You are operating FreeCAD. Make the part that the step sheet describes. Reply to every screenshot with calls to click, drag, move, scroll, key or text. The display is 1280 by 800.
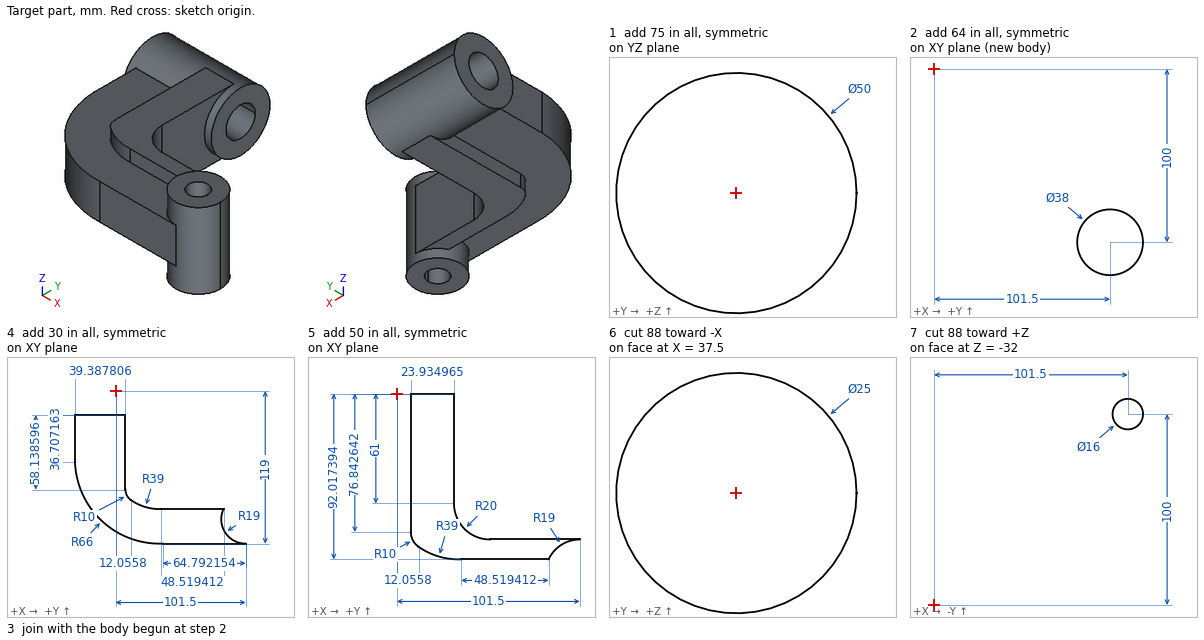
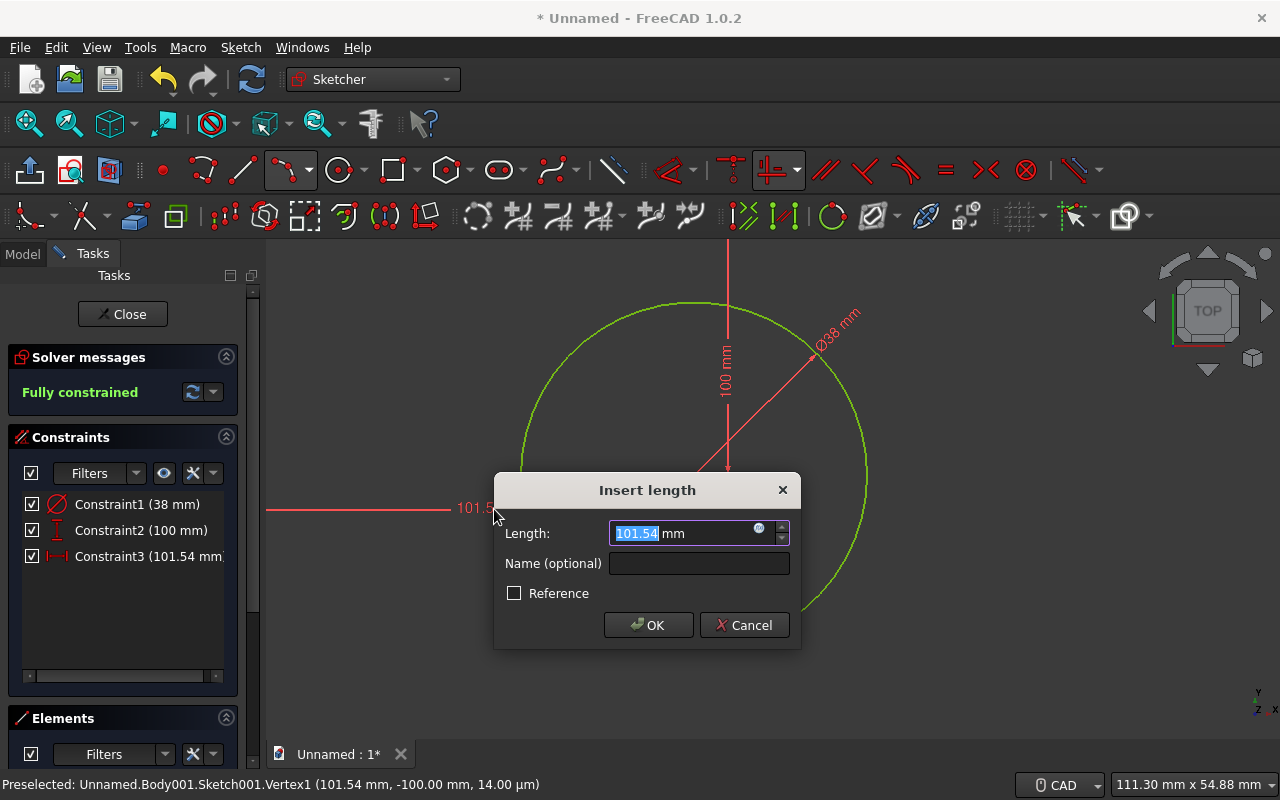
text(101.5)
key(Return)
key(Escape)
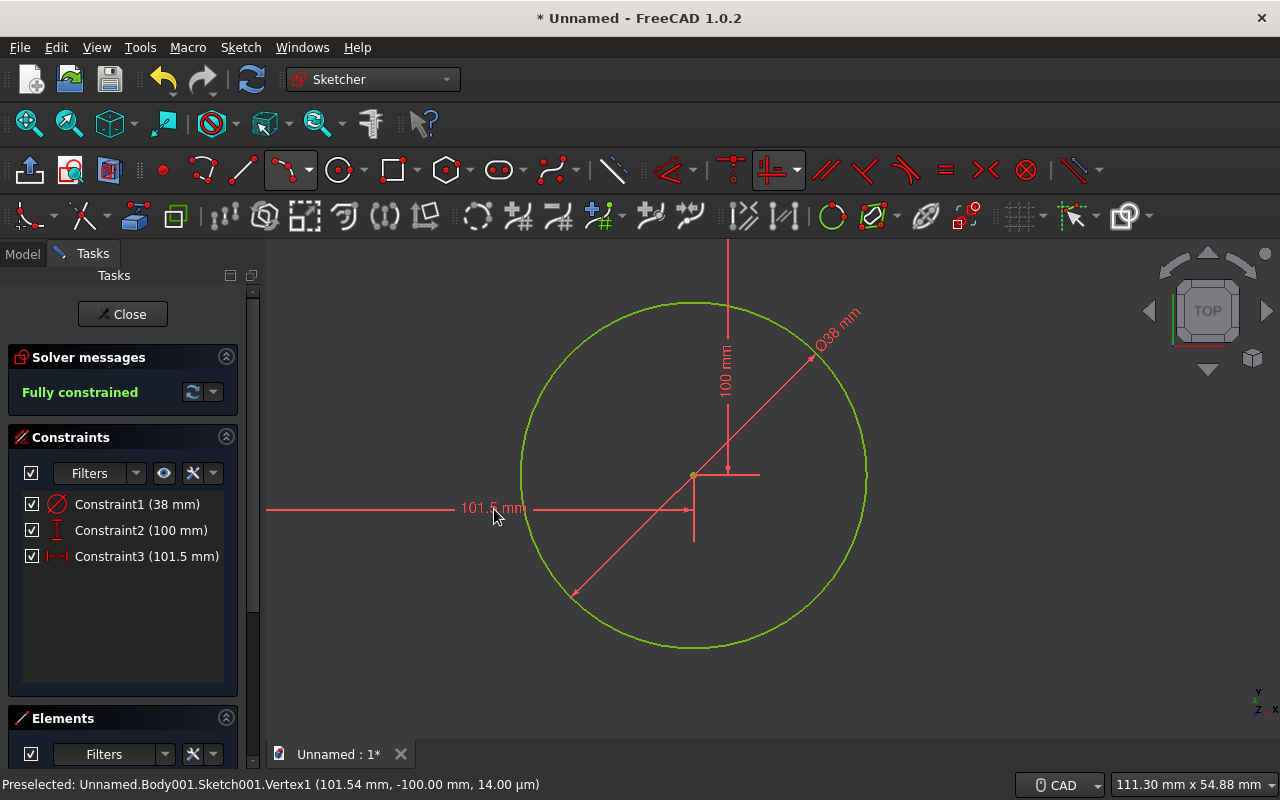
click(123, 314)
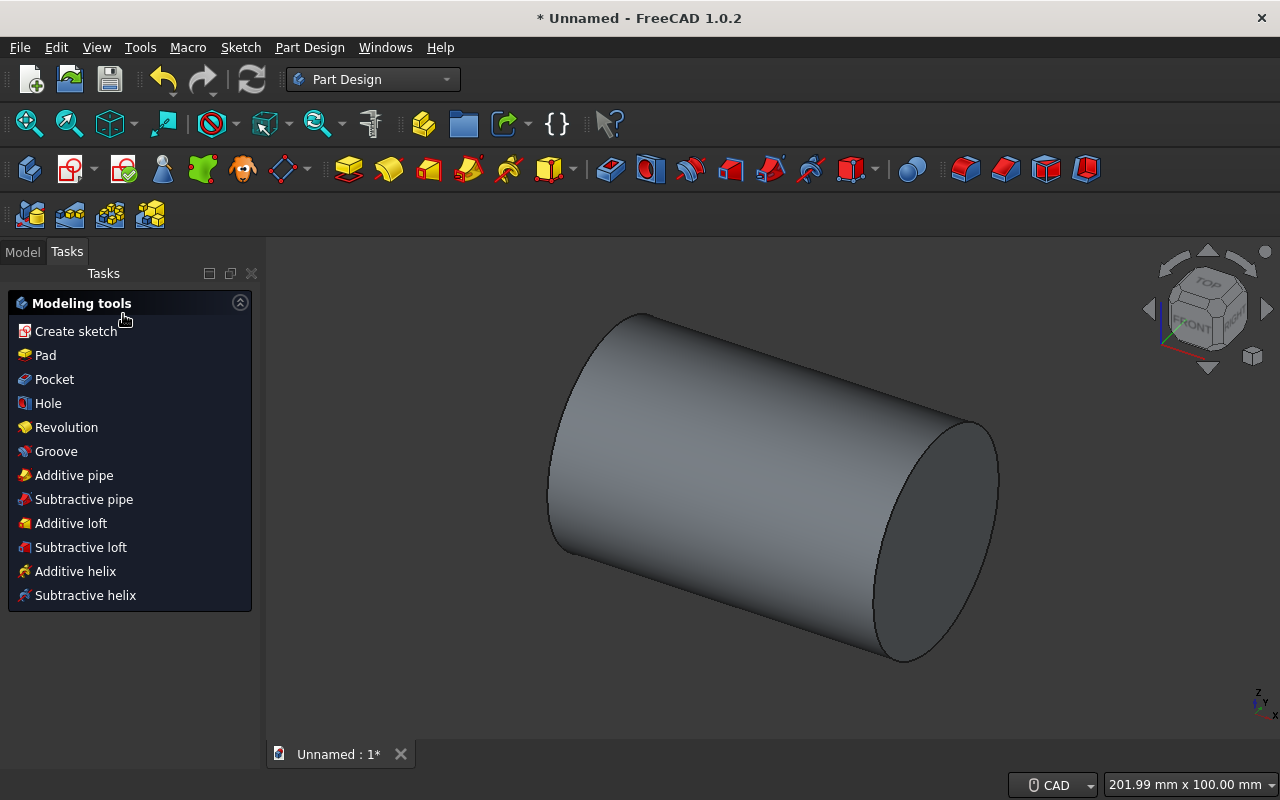
click(350, 170)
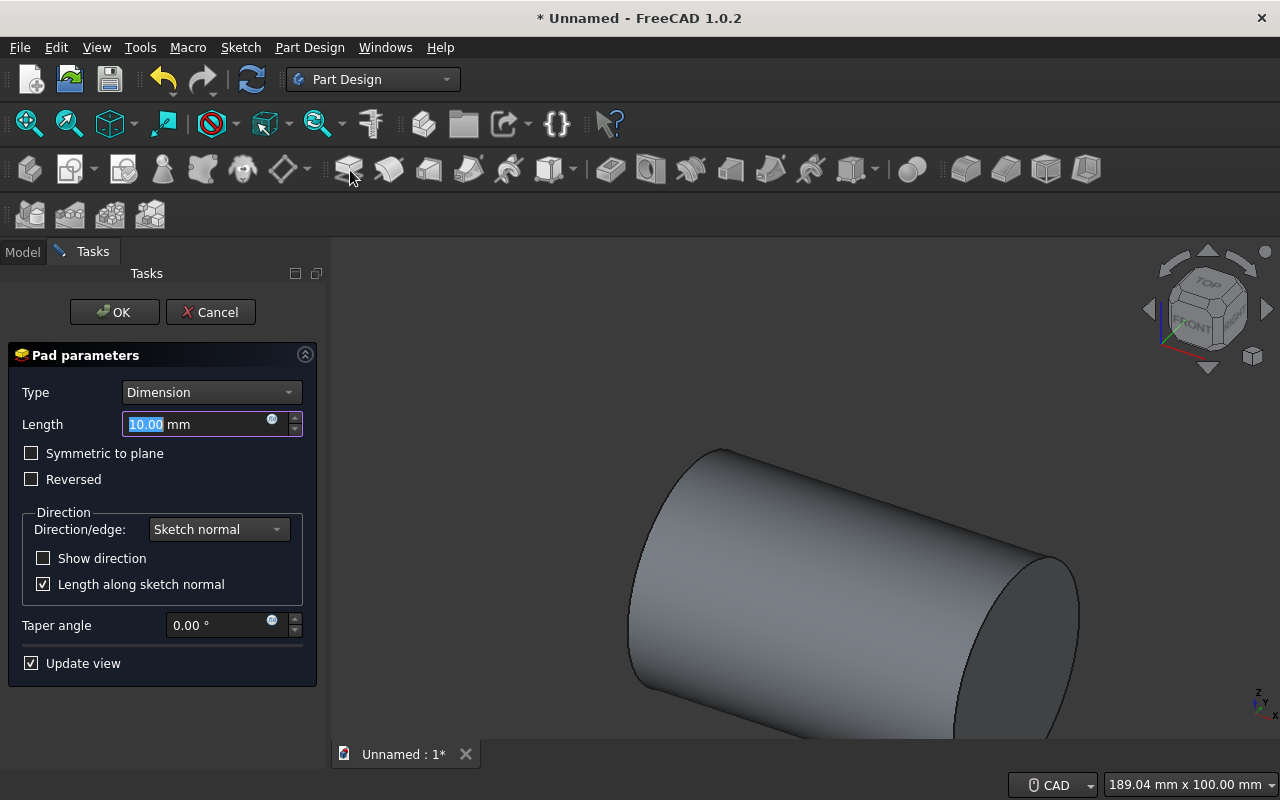
text(64)
key(Tab)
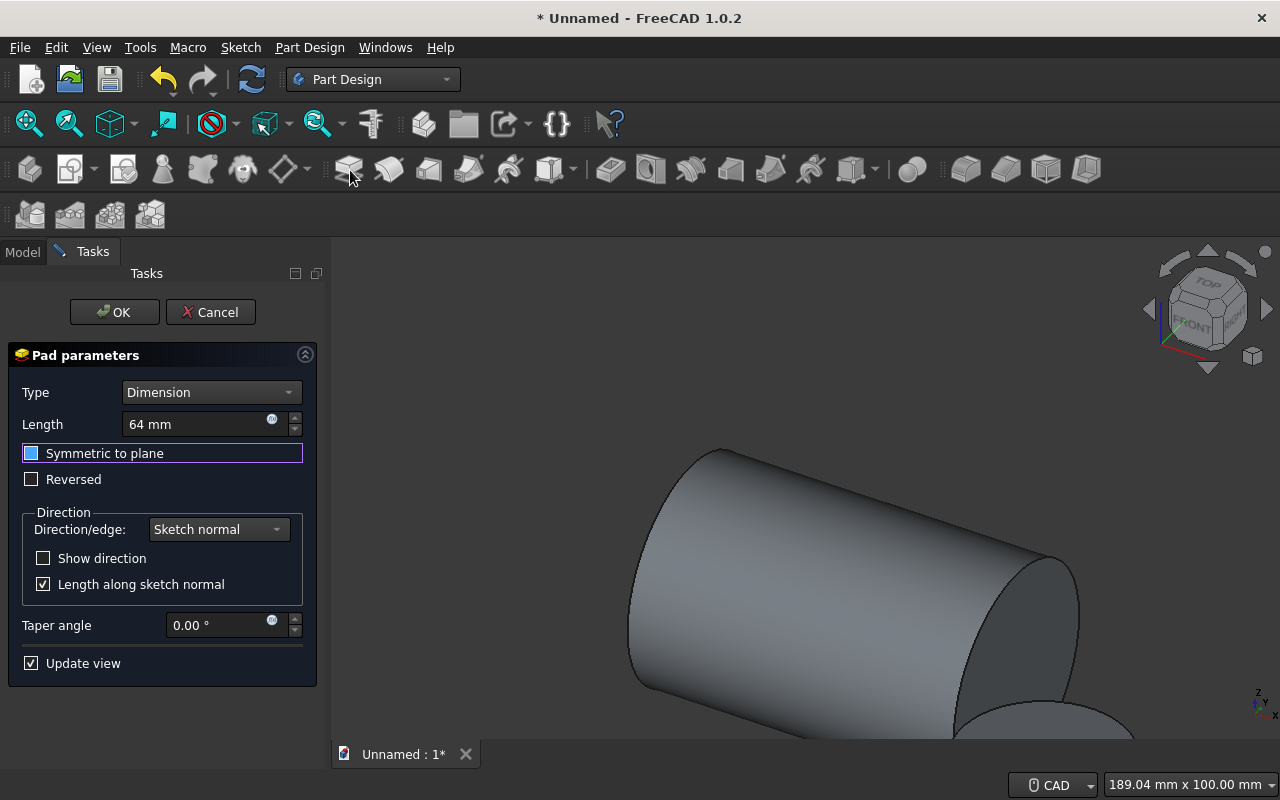
click(30, 453)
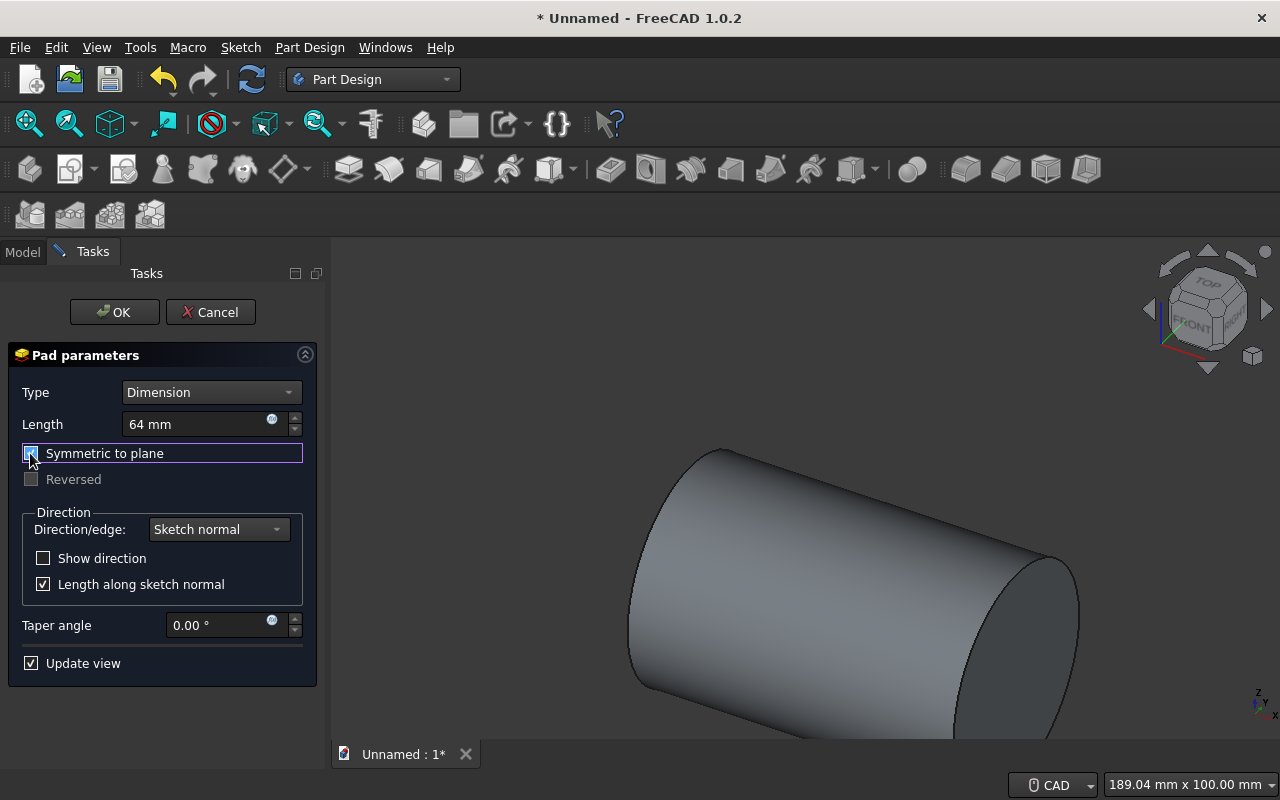
click(115, 312)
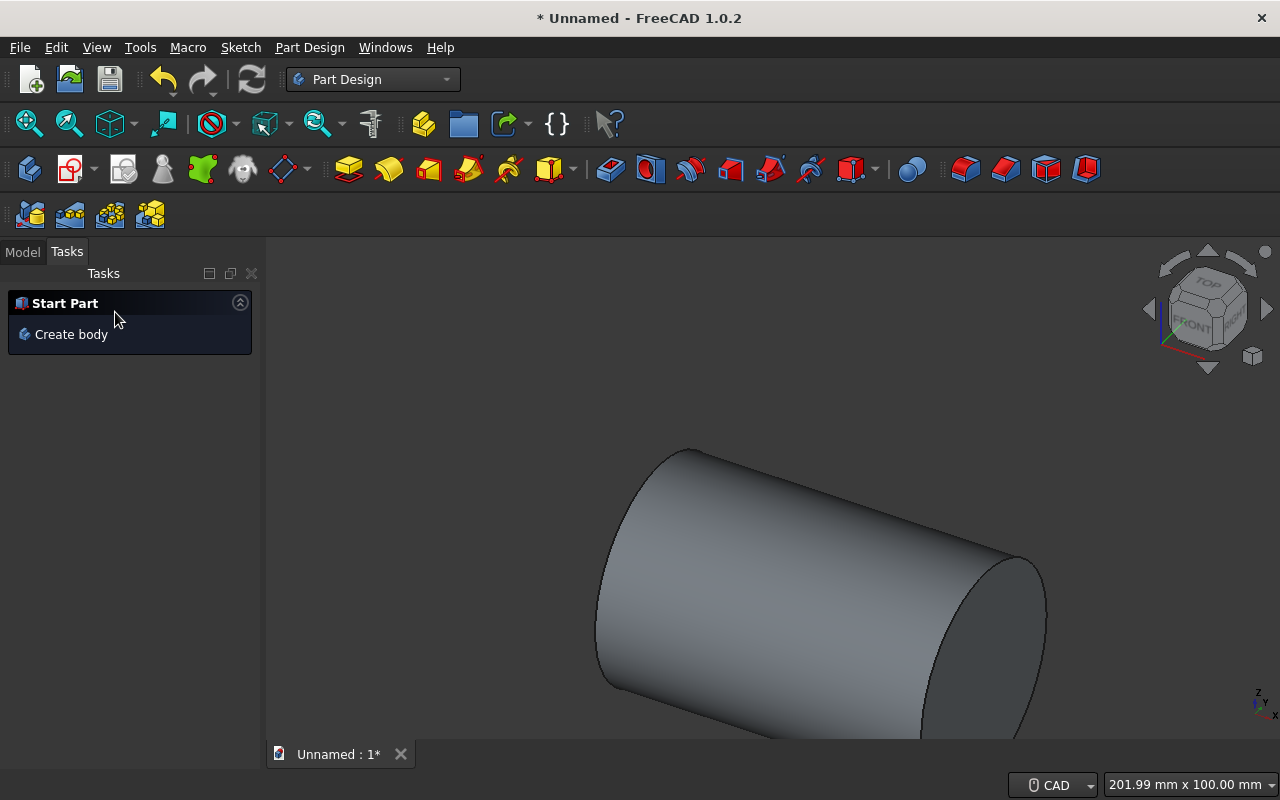
key(v)
key(f)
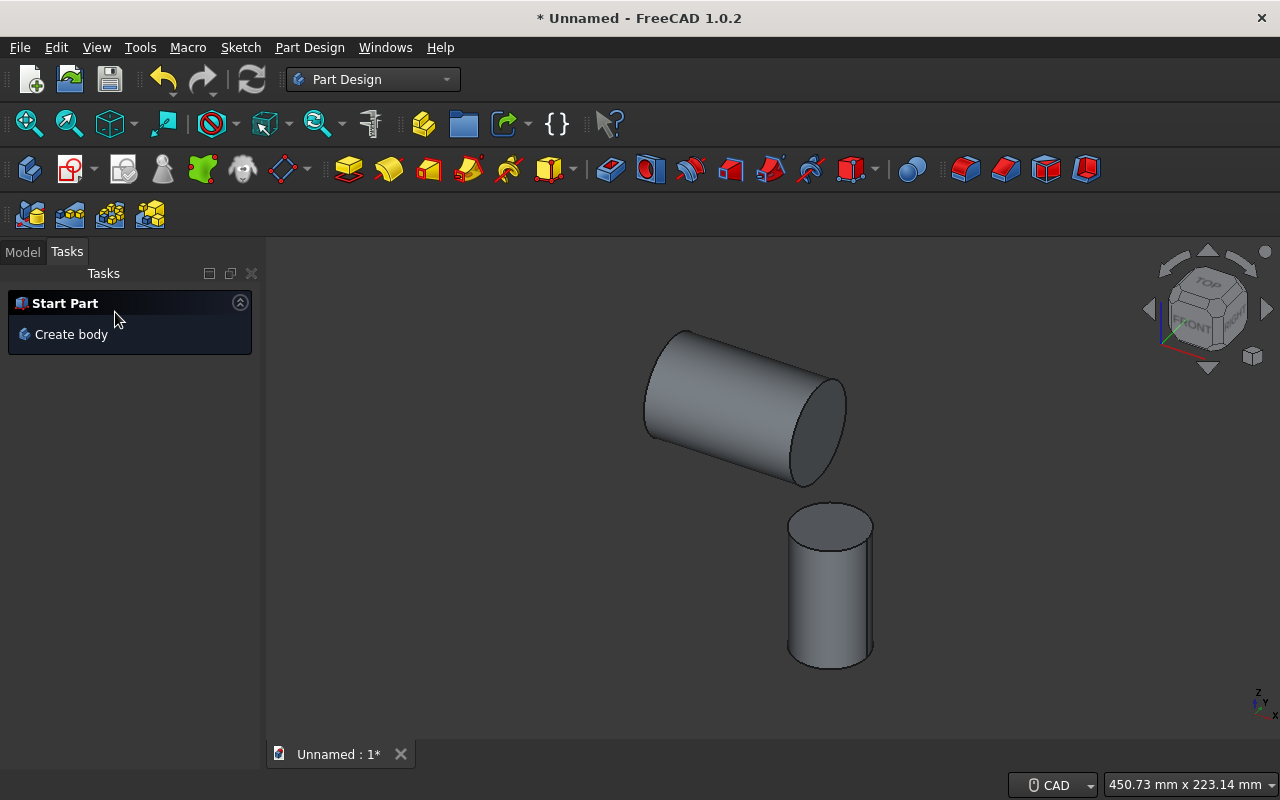
click(23, 251)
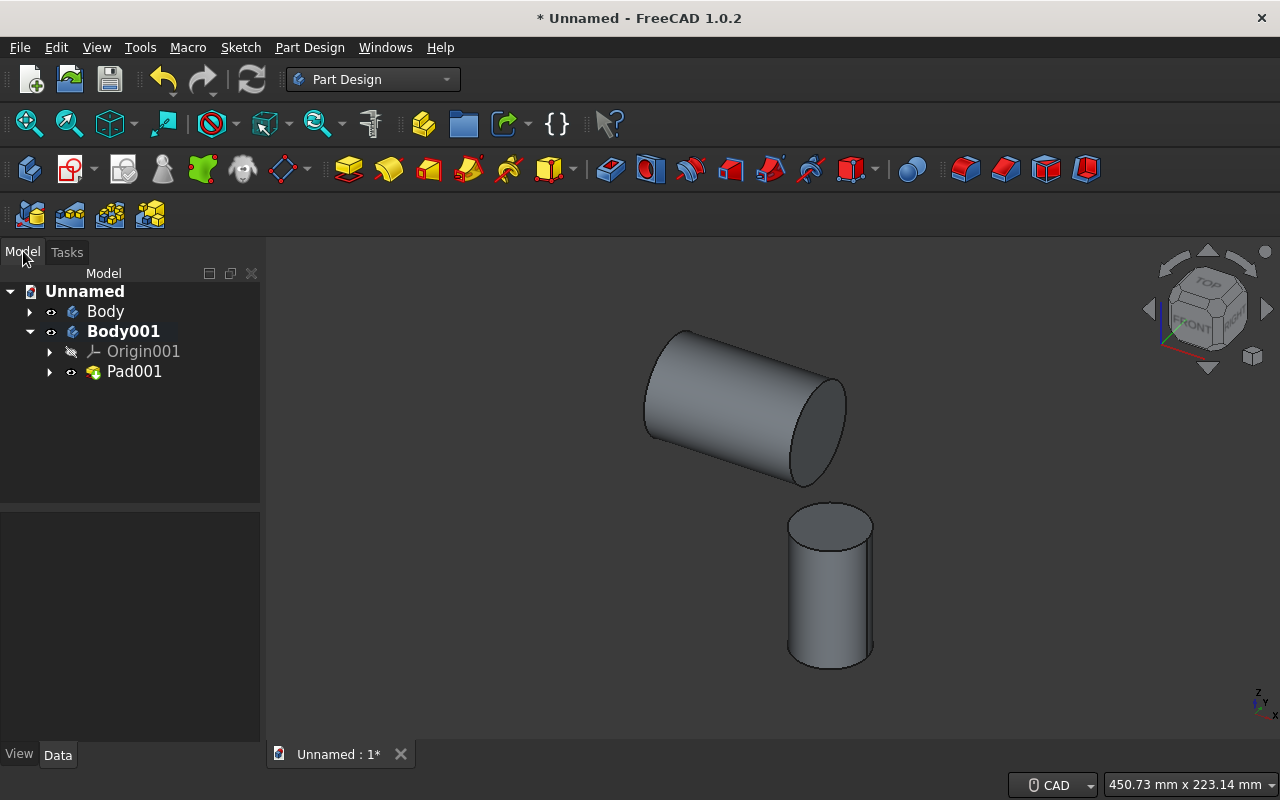
double_click(96, 312)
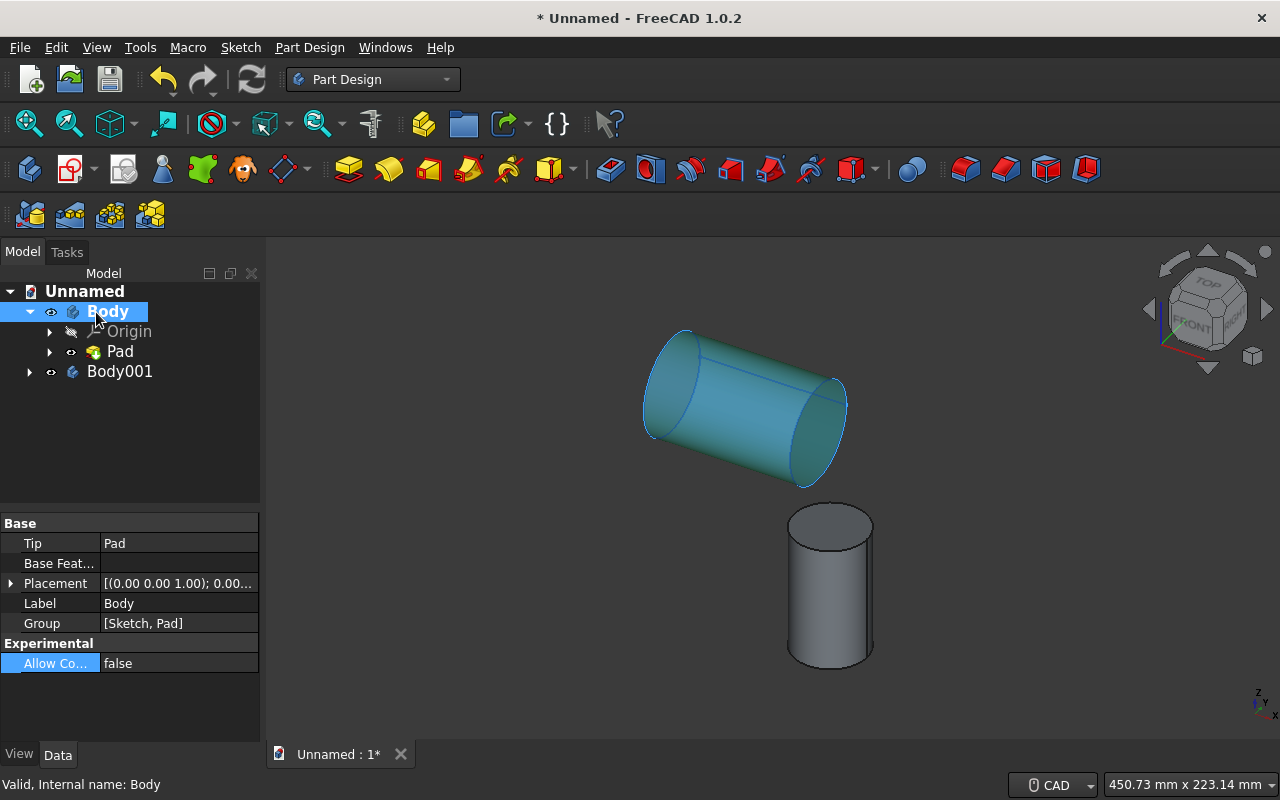
click(96, 312)